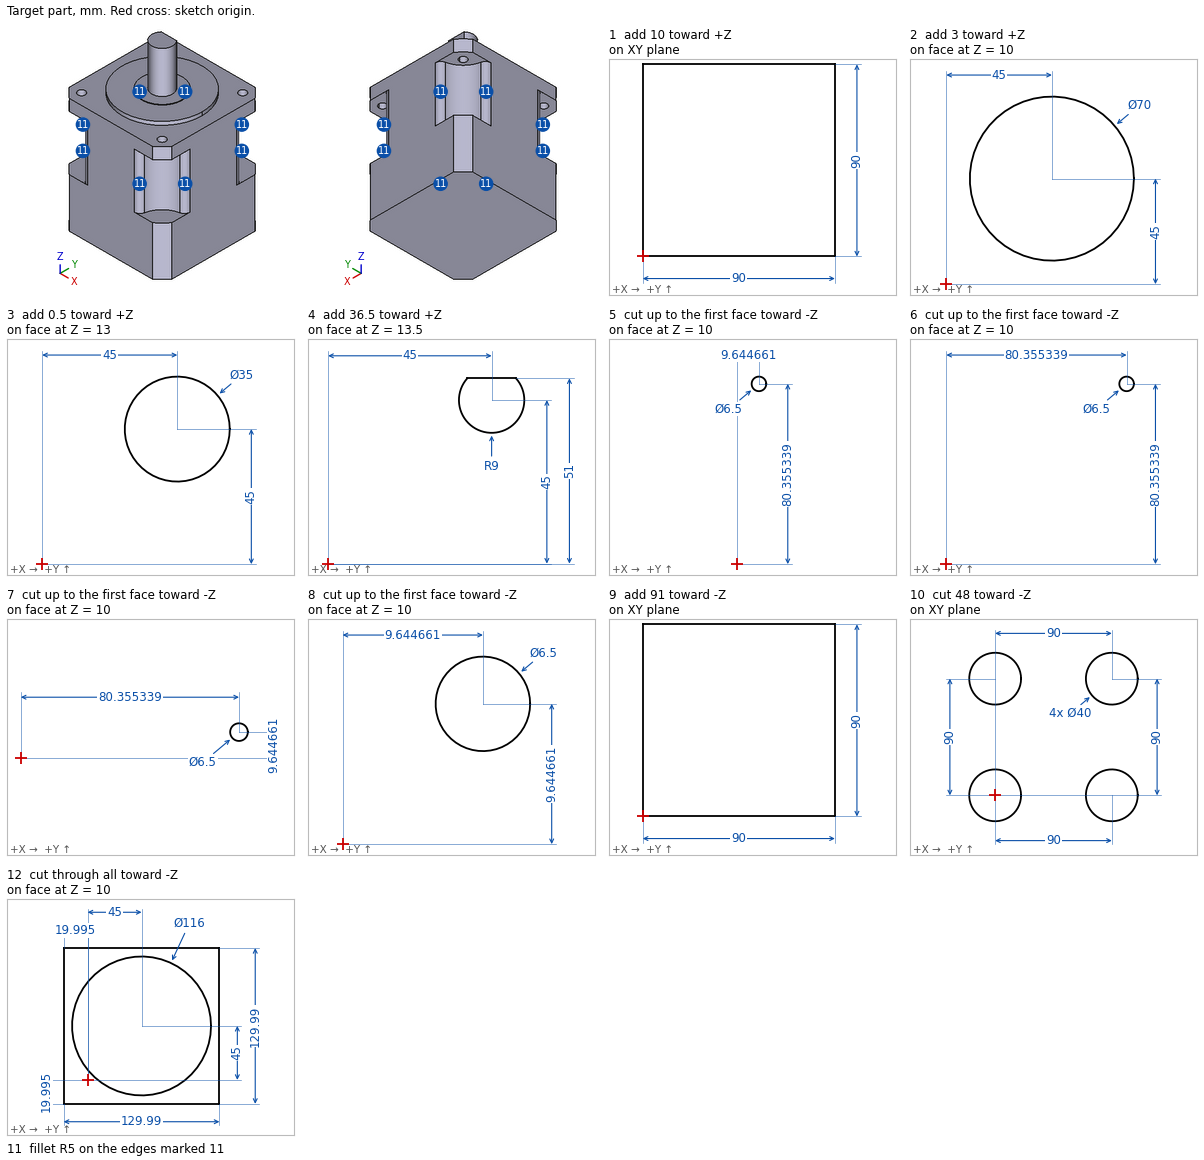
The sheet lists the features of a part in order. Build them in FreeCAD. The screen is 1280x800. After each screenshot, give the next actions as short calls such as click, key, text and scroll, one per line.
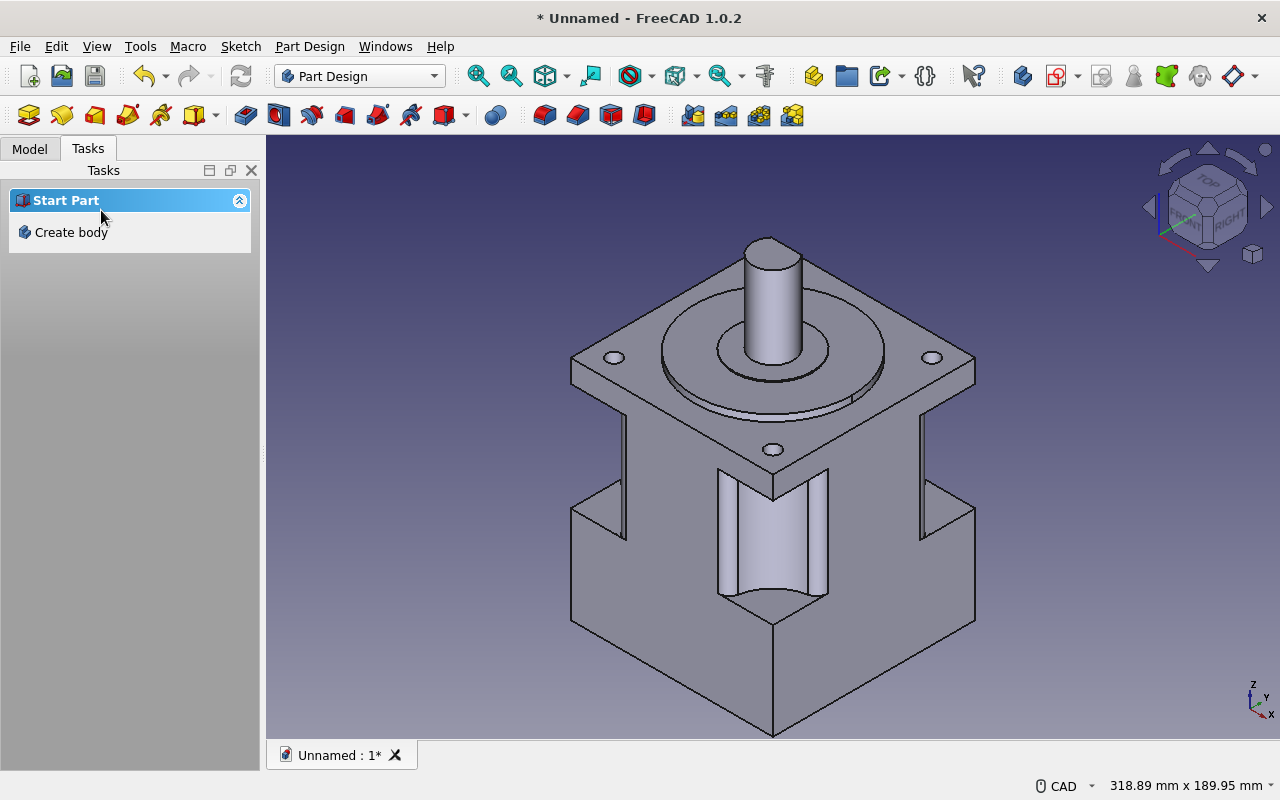
click(918, 374)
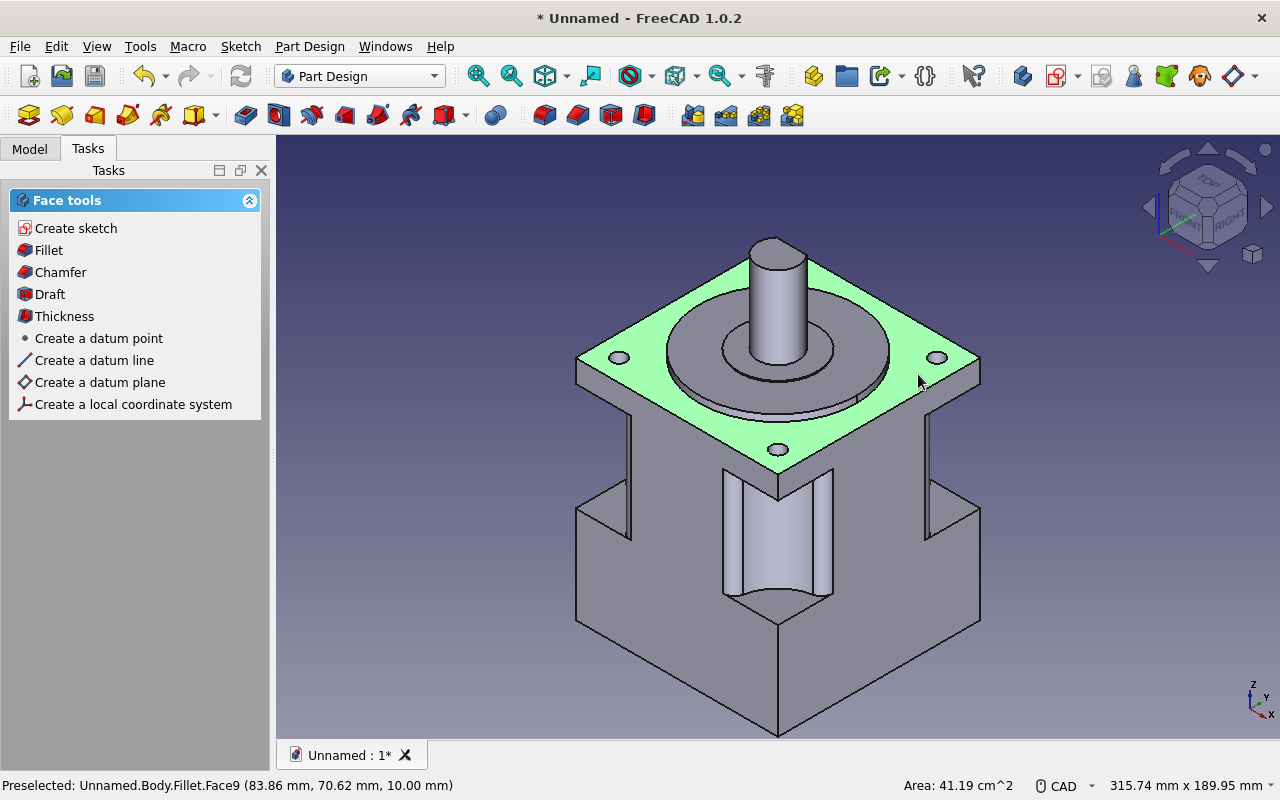
click(1056, 76)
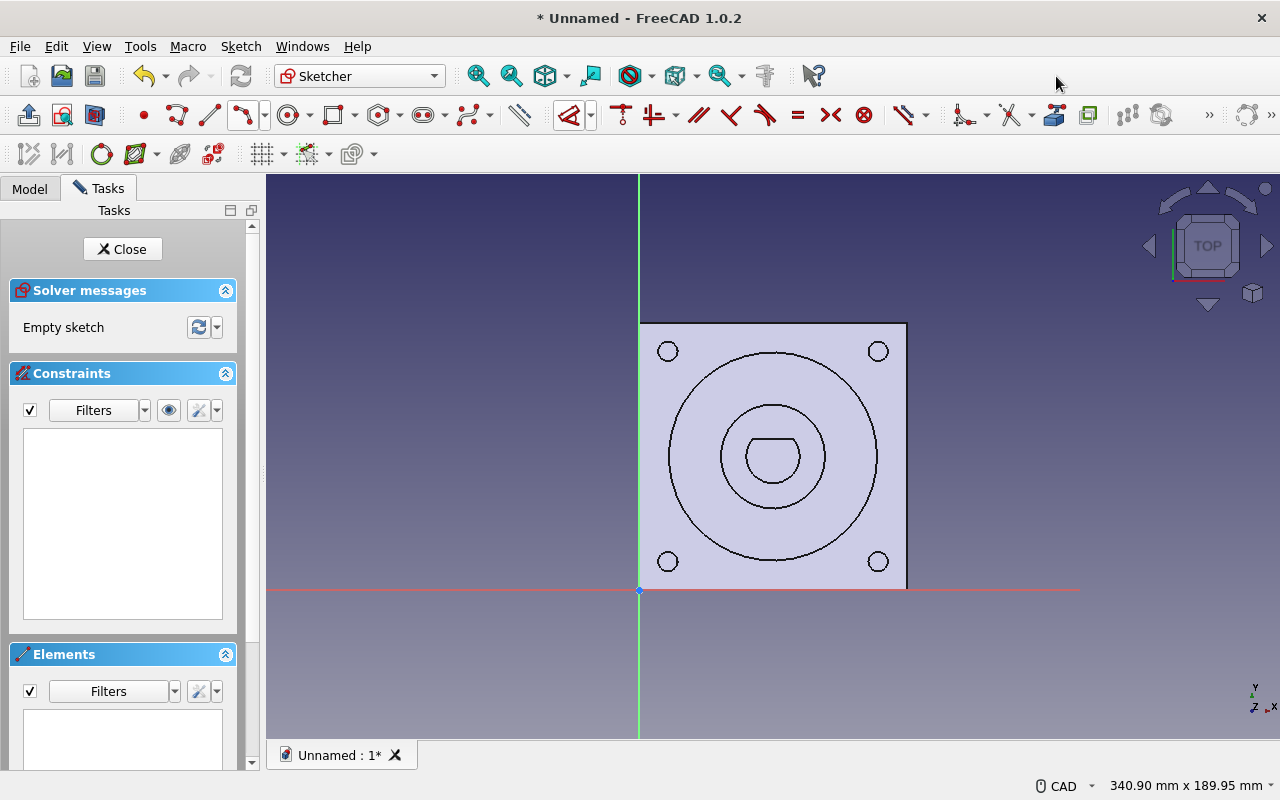
key(q)
key(s)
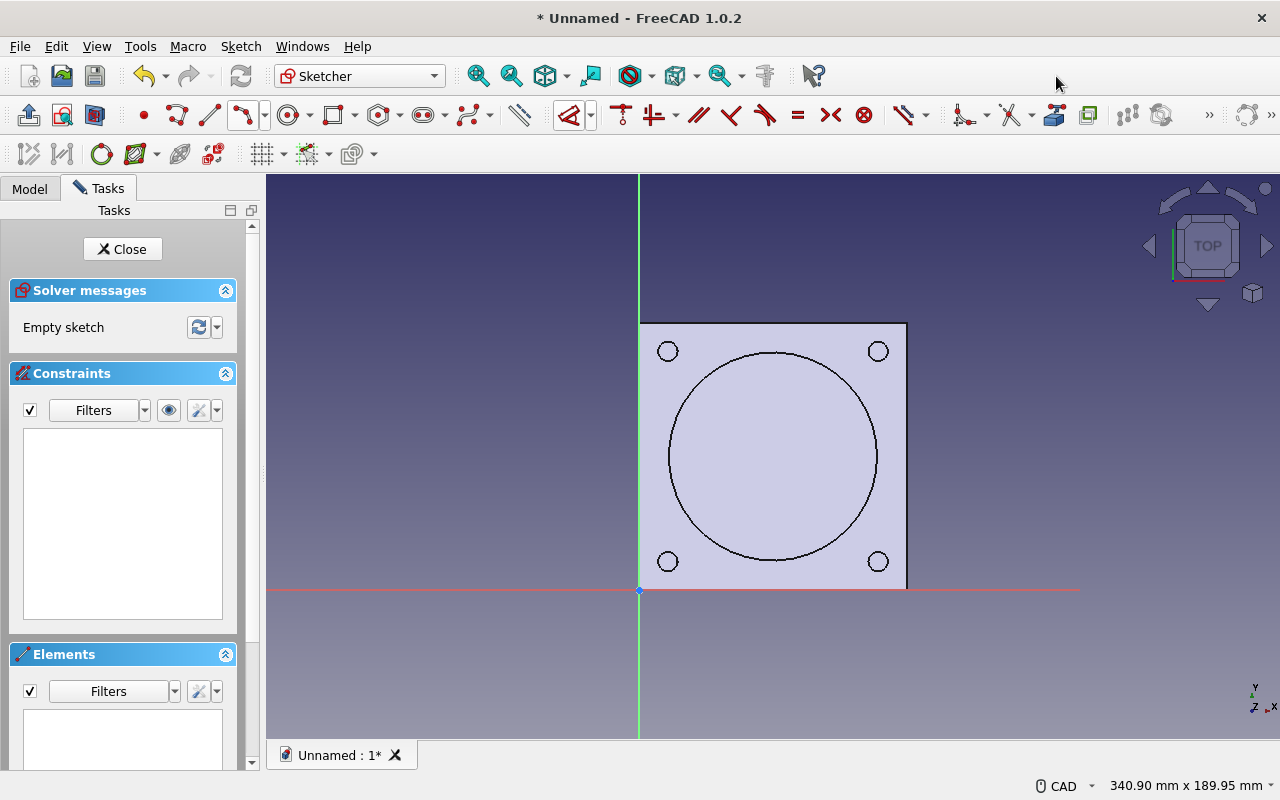
key(g)
key(r)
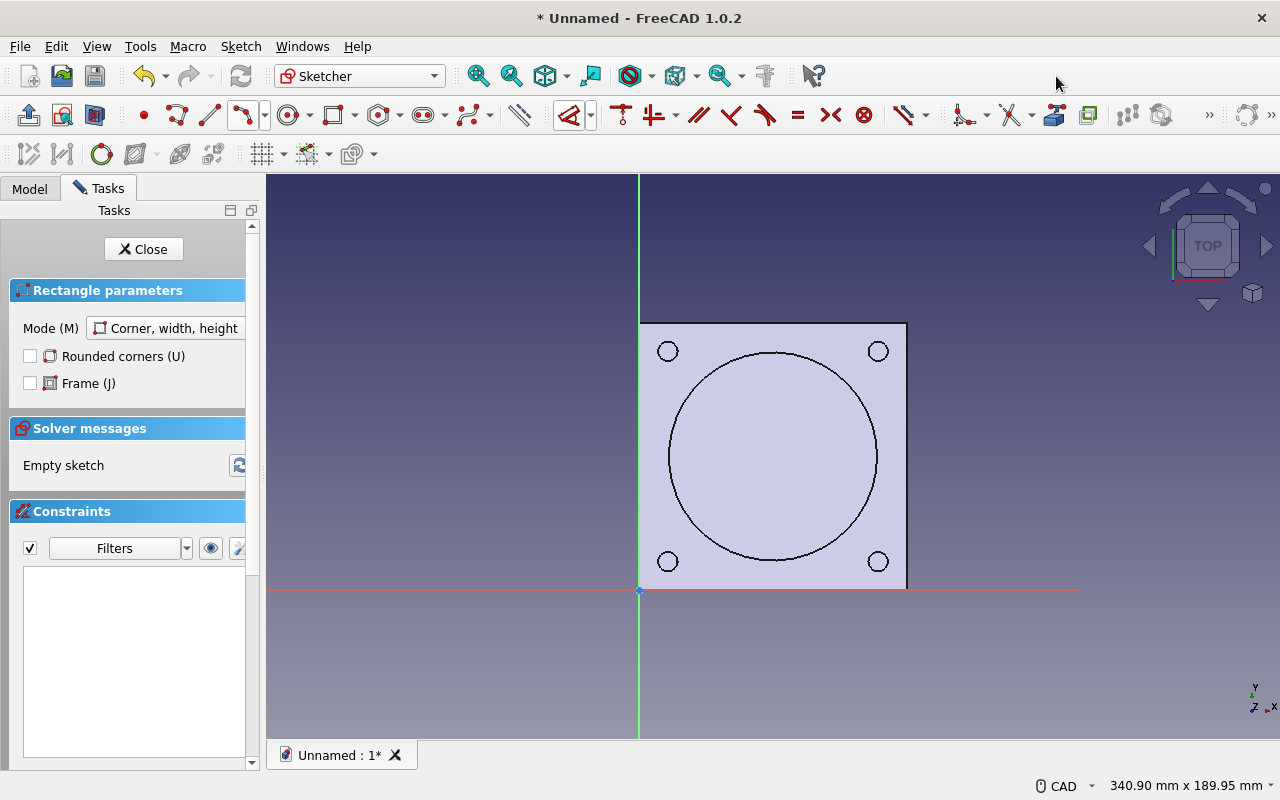
click(580, 263)
move(966, 650)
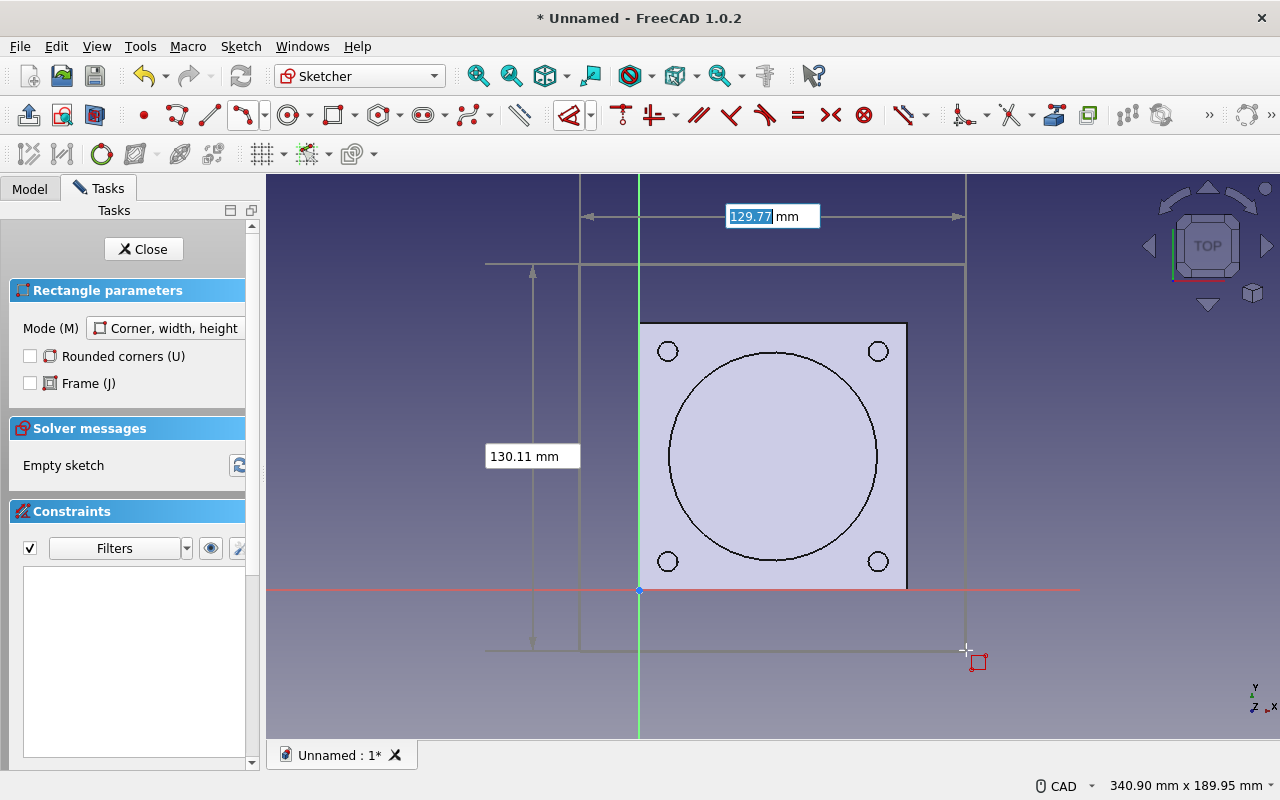
text(129.99)
key(Tab)
text(129.99)
key(Return)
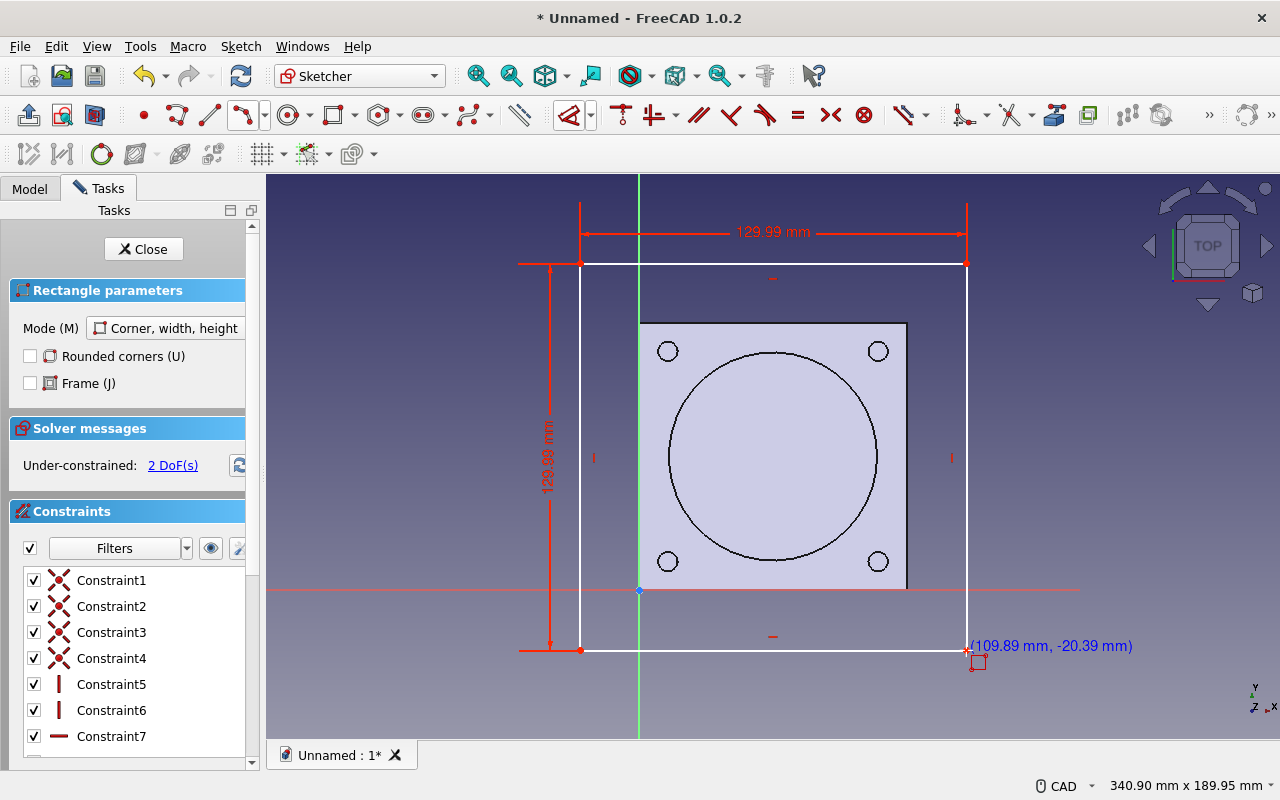
key(g)
key(c)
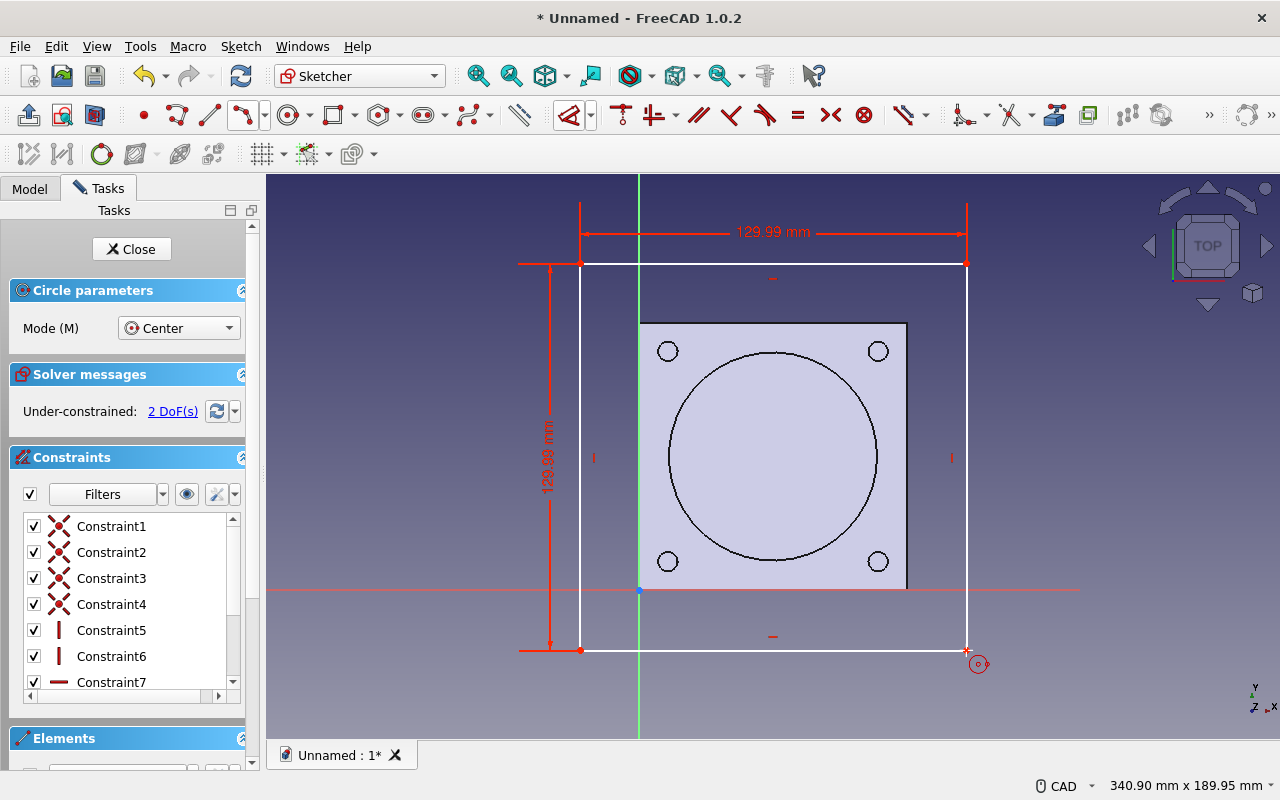
click(773, 457)
move(895, 335)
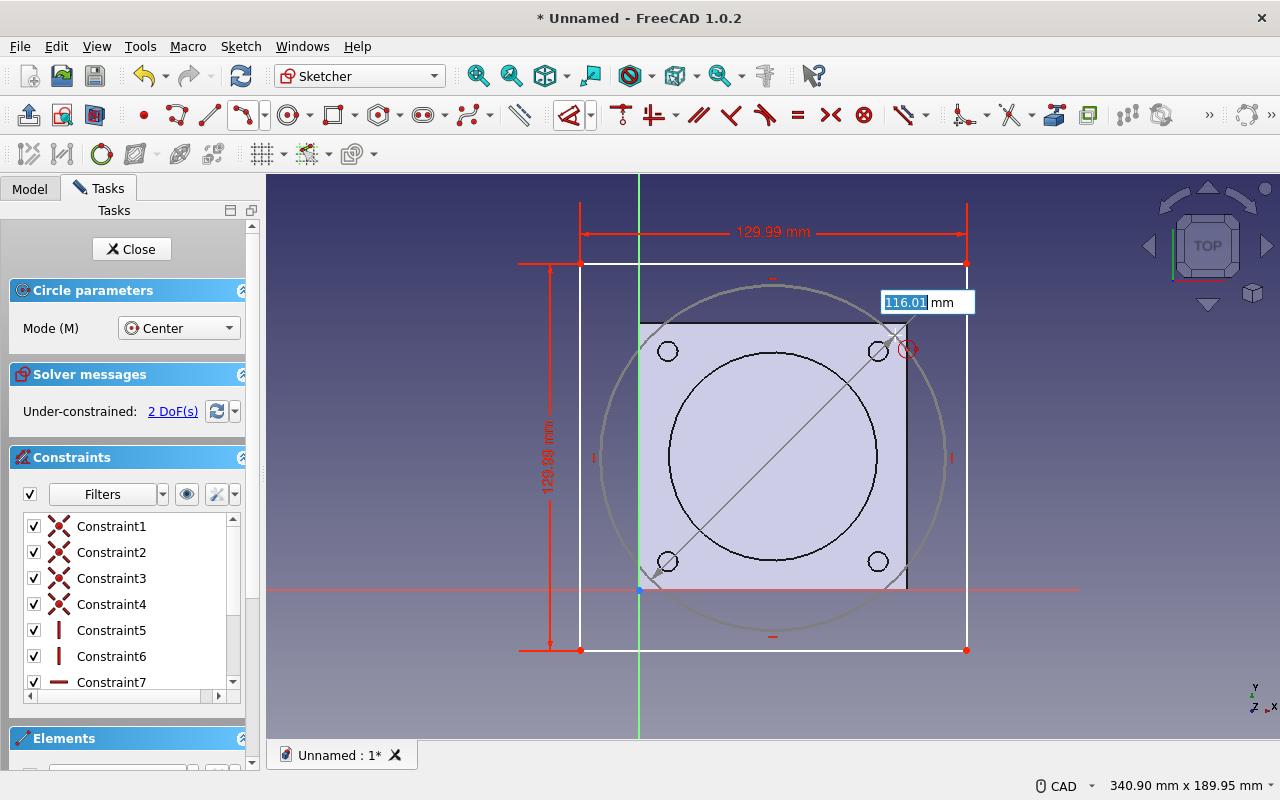
text(116)
key(Return)
key(Escape)